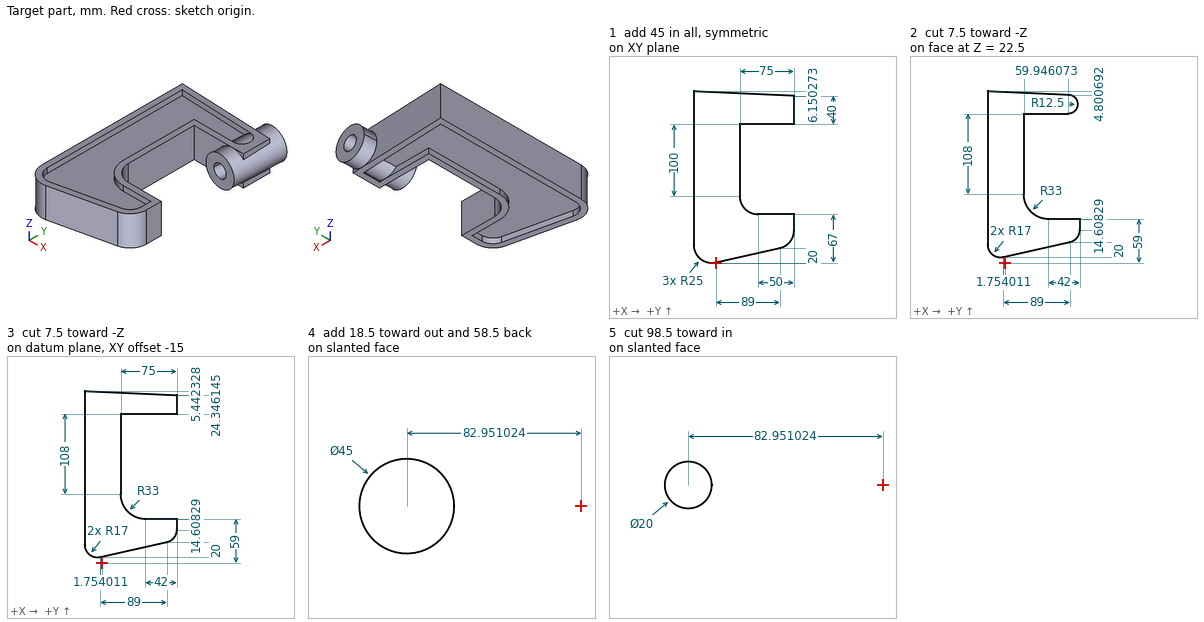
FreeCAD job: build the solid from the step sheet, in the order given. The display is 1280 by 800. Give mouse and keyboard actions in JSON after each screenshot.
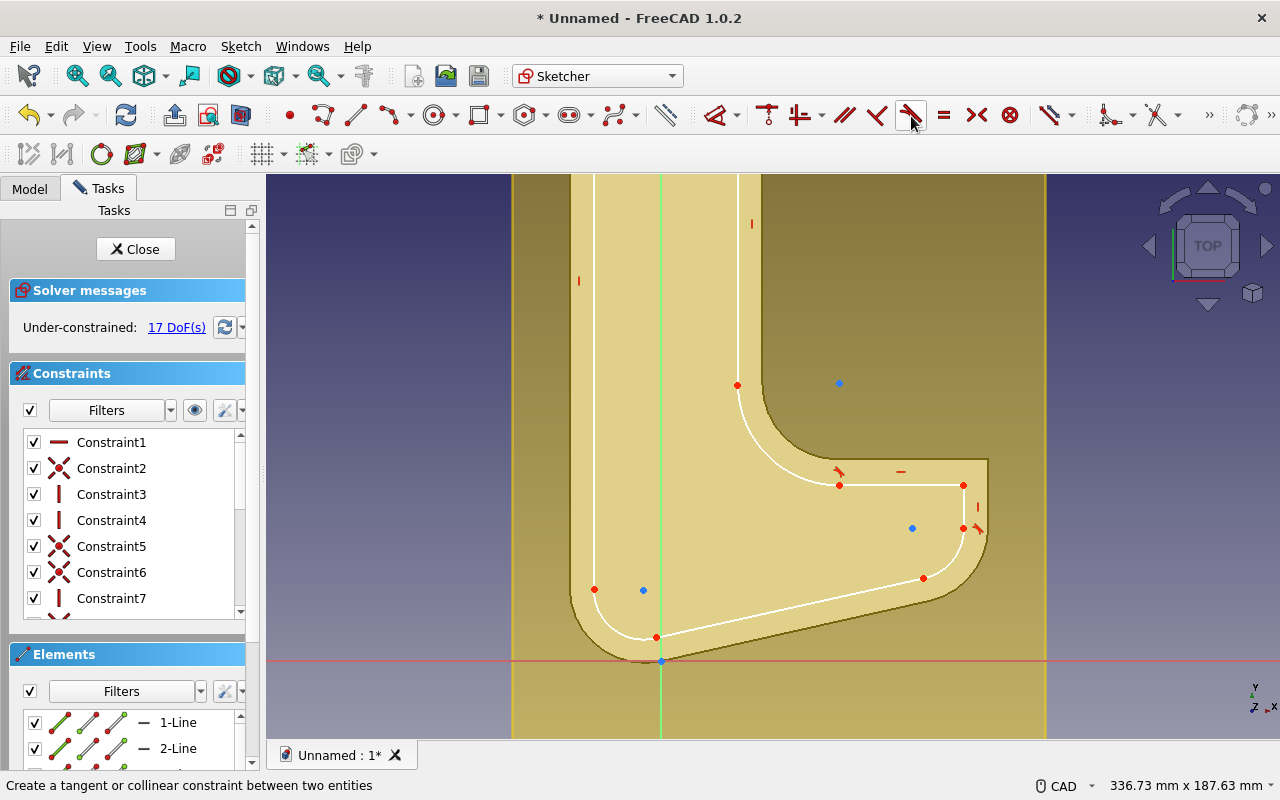
{"action": "left_click", "coordinate": [844, 596]}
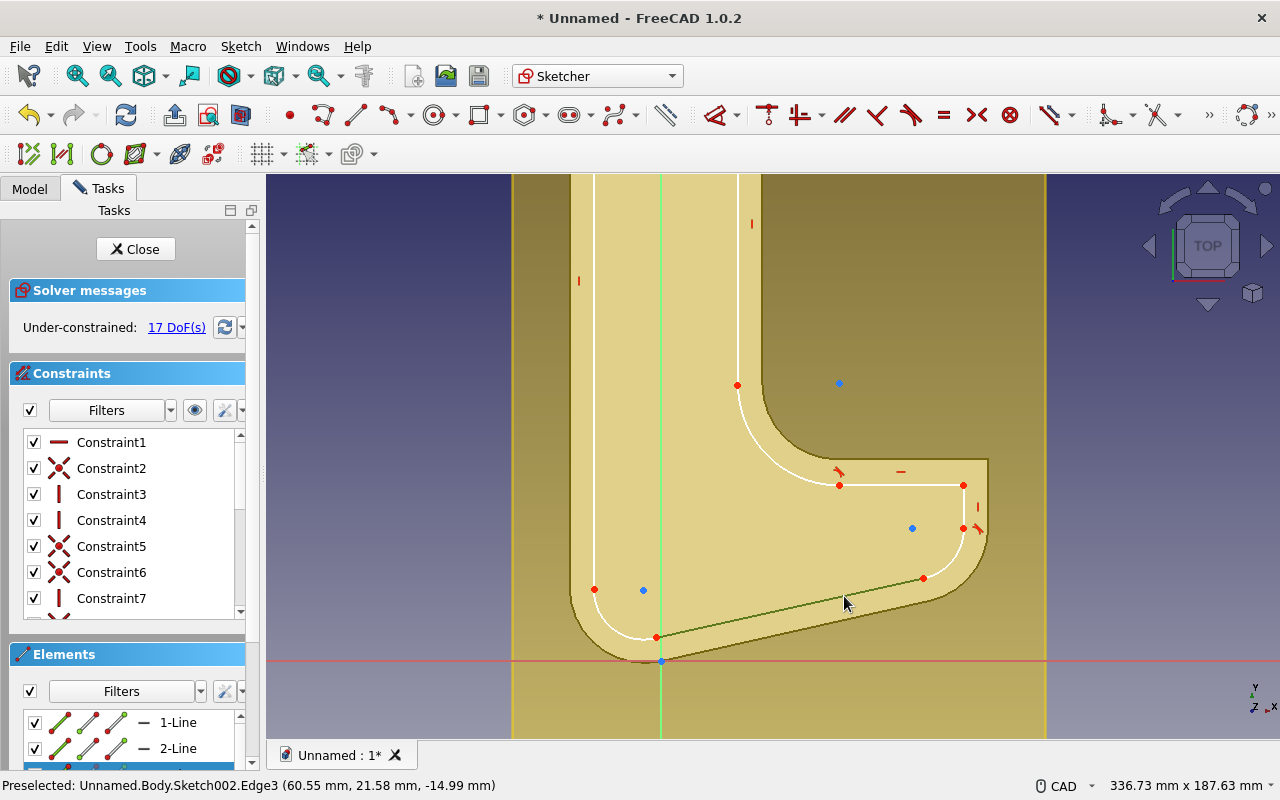
{"action": "left_click", "coordinate": [943, 570]}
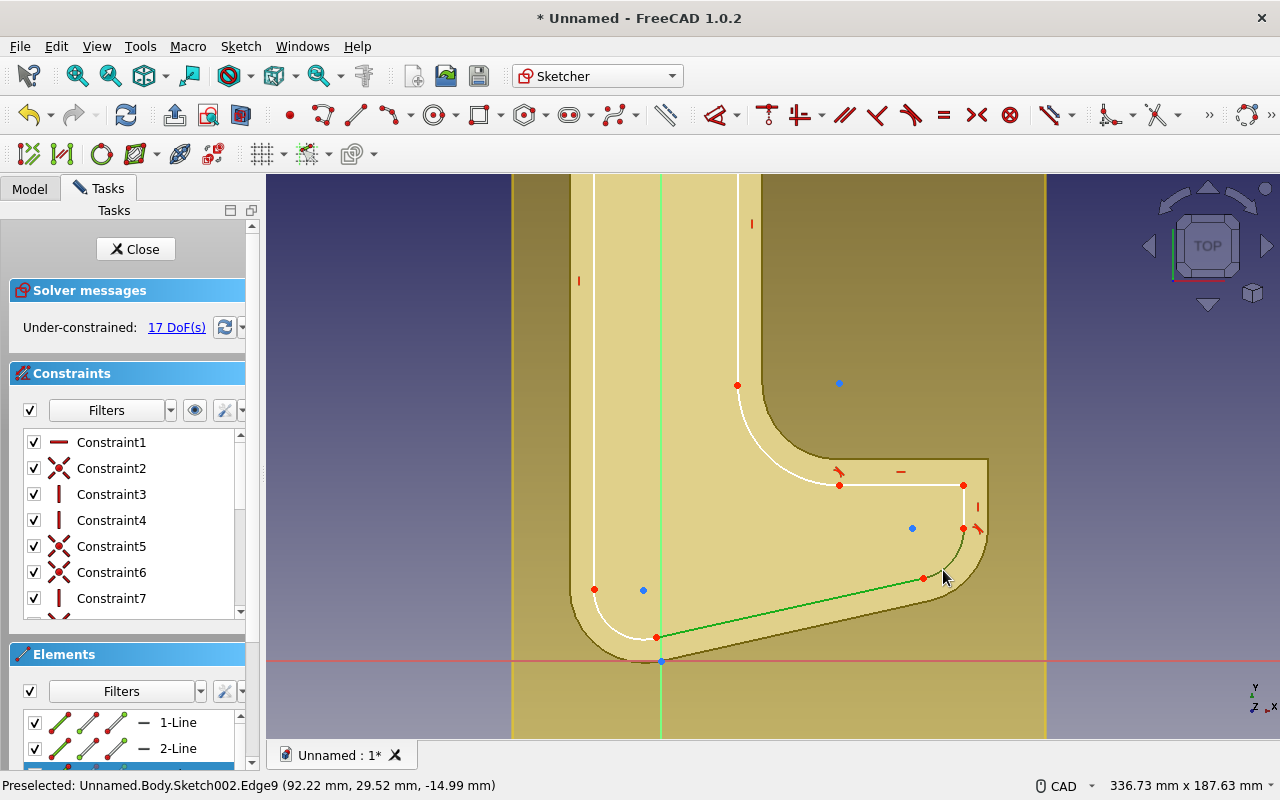
{"action": "left_click", "coordinate": [911, 116]}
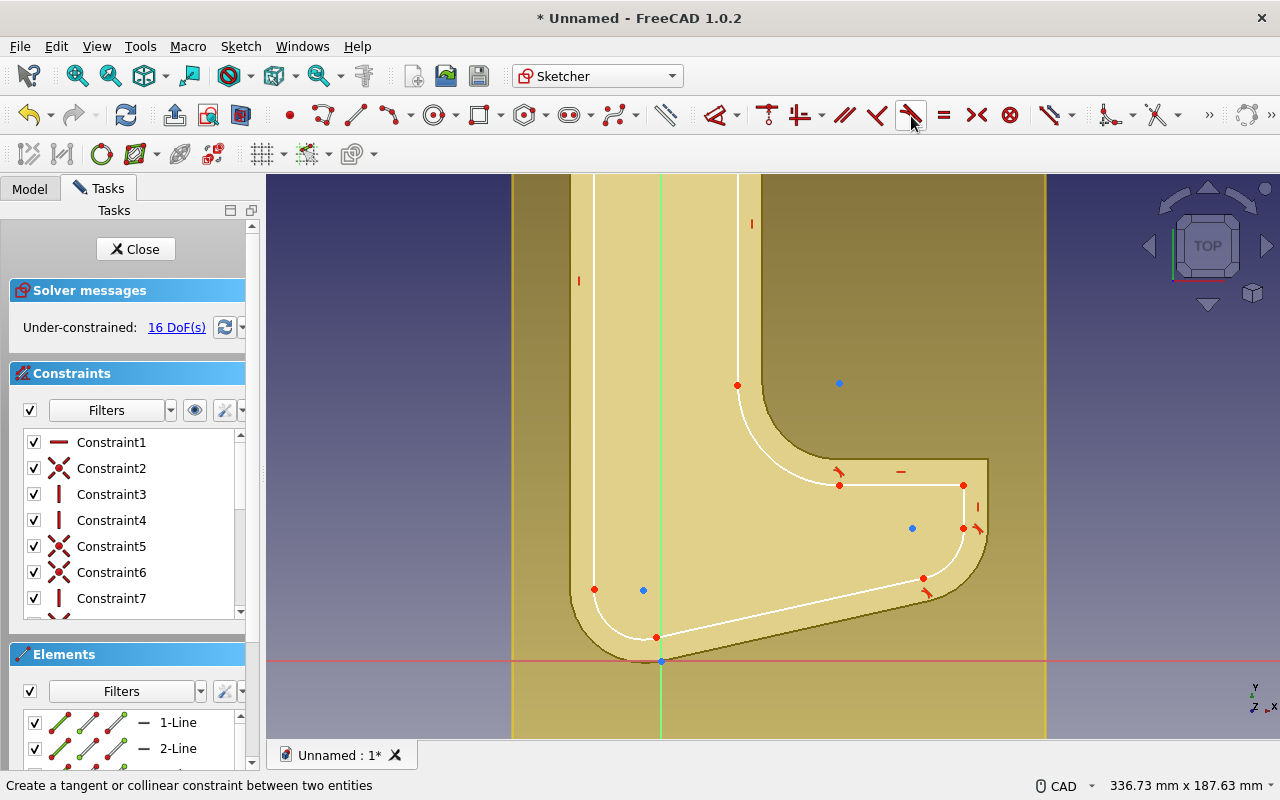
{"action": "left_click", "coordinate": [844, 596]}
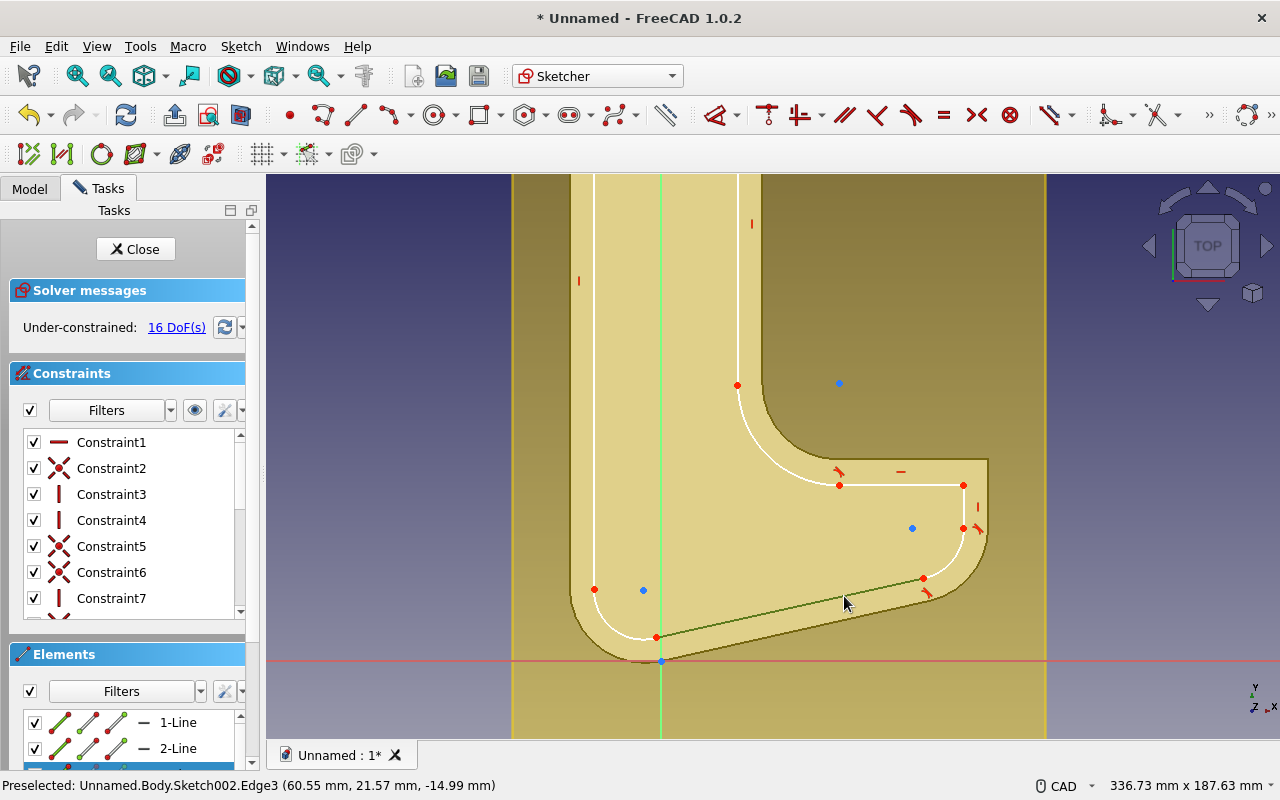
{"action": "left_click", "coordinate": [601, 616]}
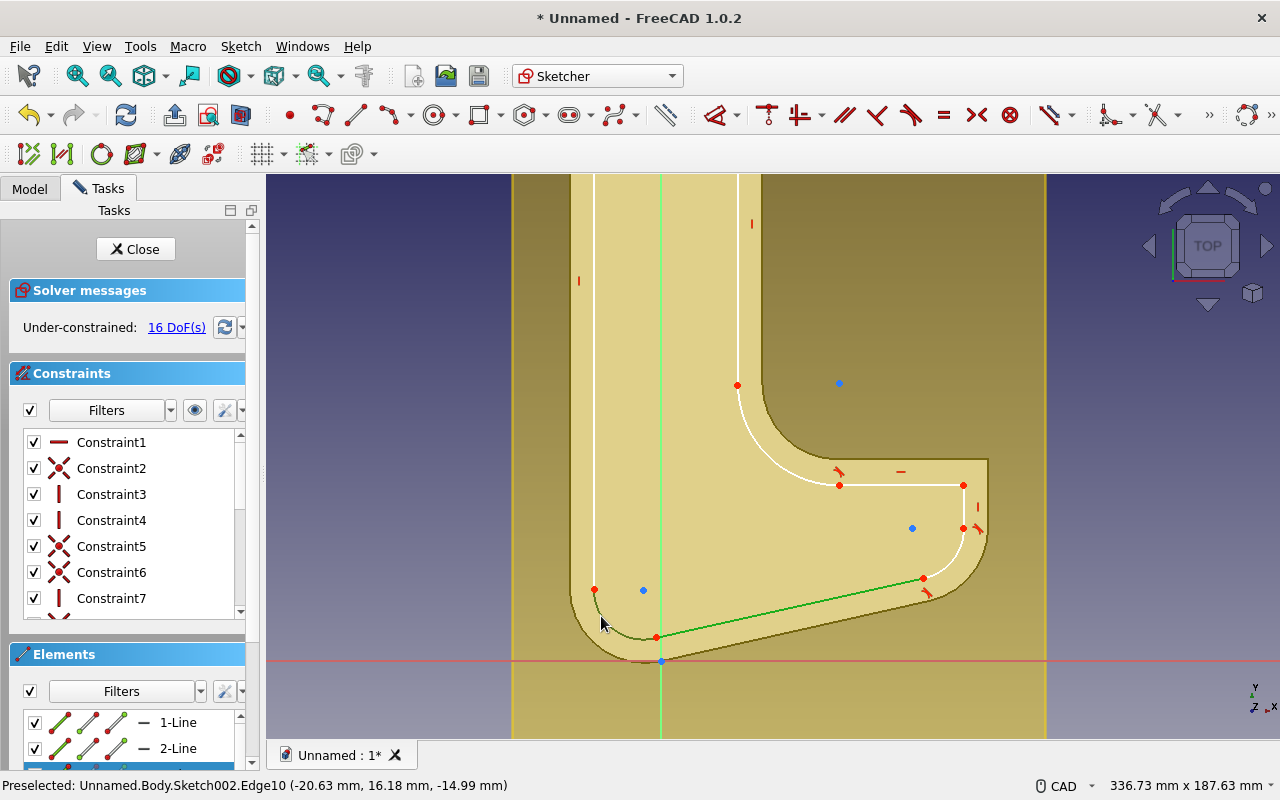
{"action": "left_click", "coordinate": [911, 116]}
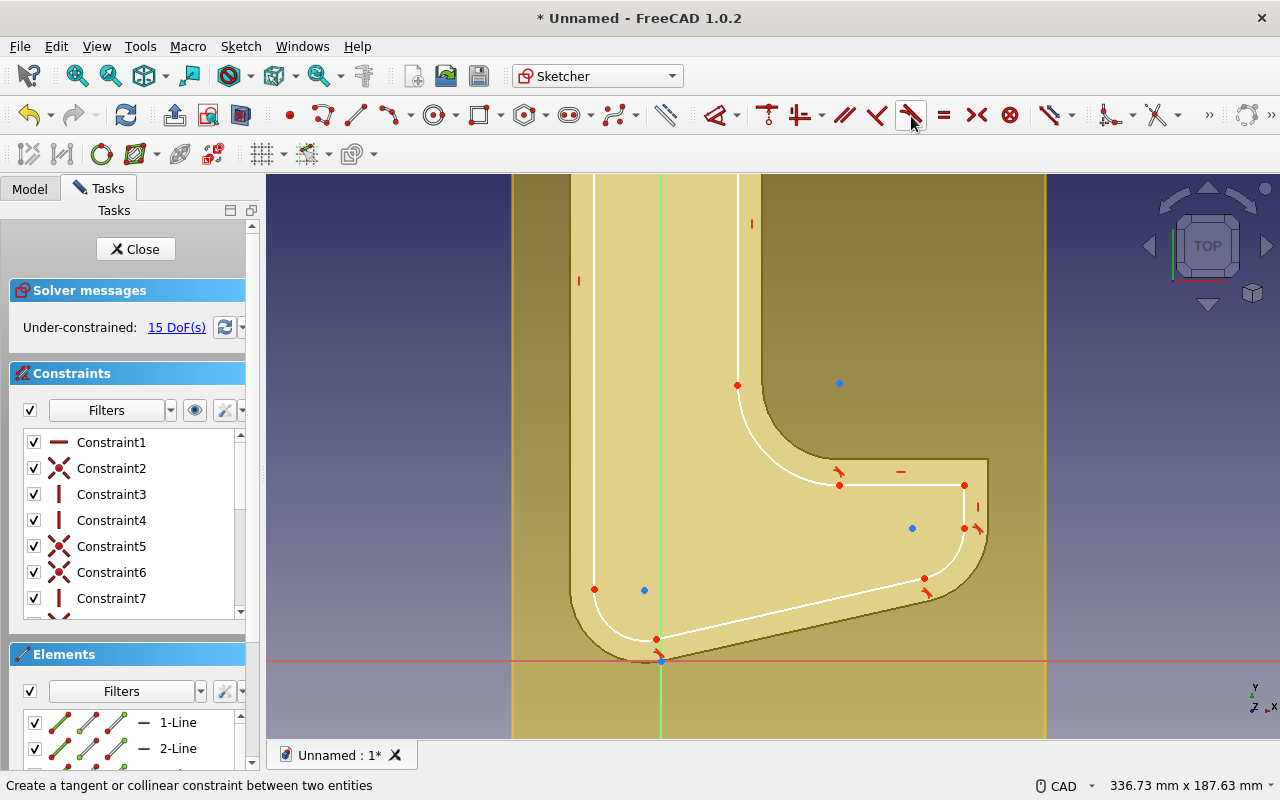
{"action": "left_click", "coordinate": [594, 404]}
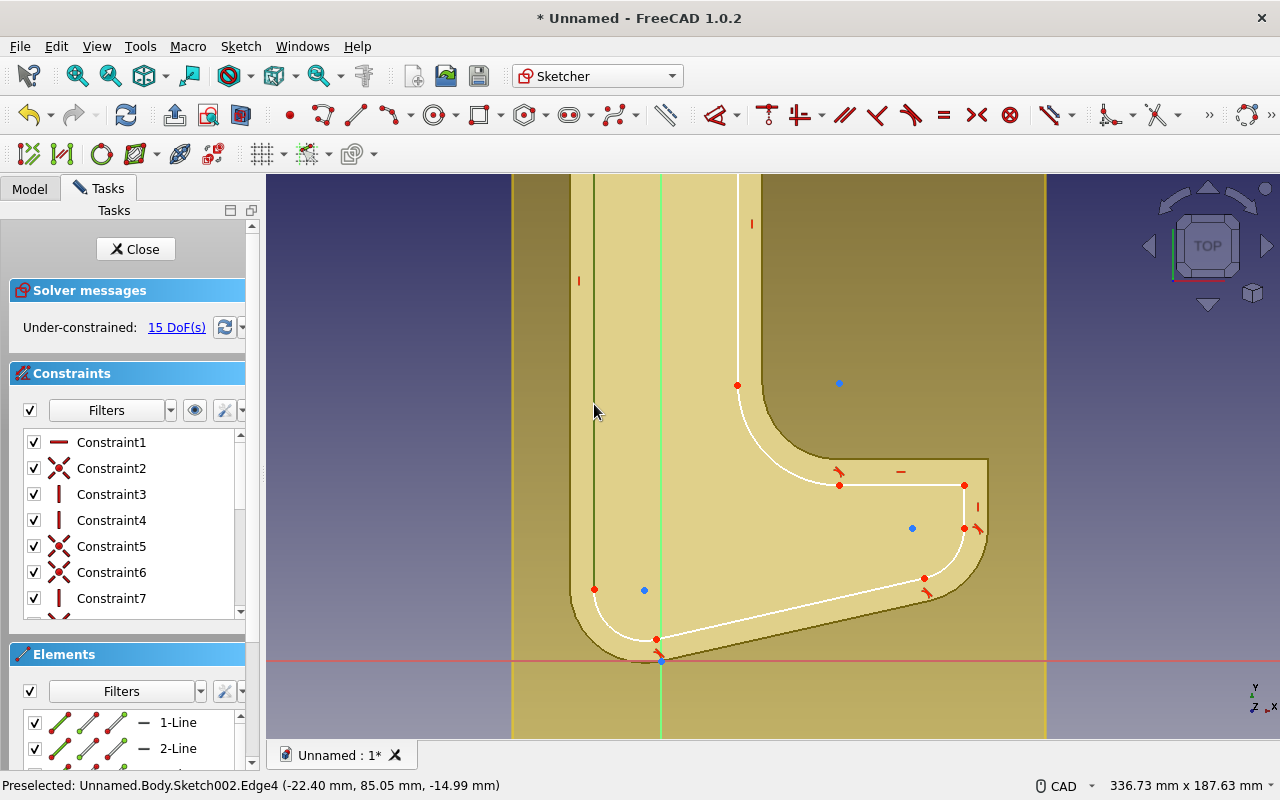
{"action": "left_click", "coordinate": [601, 616]}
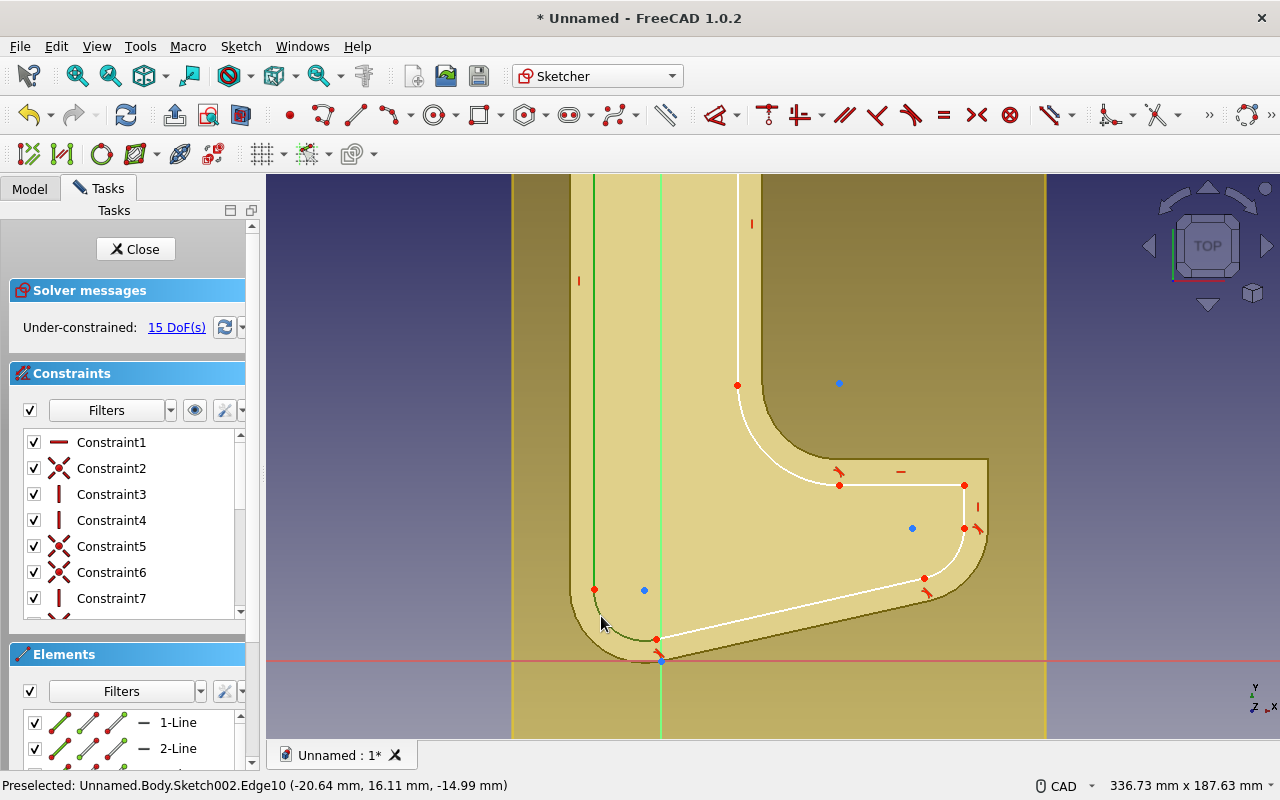
{"action": "left_click", "coordinate": [911, 116]}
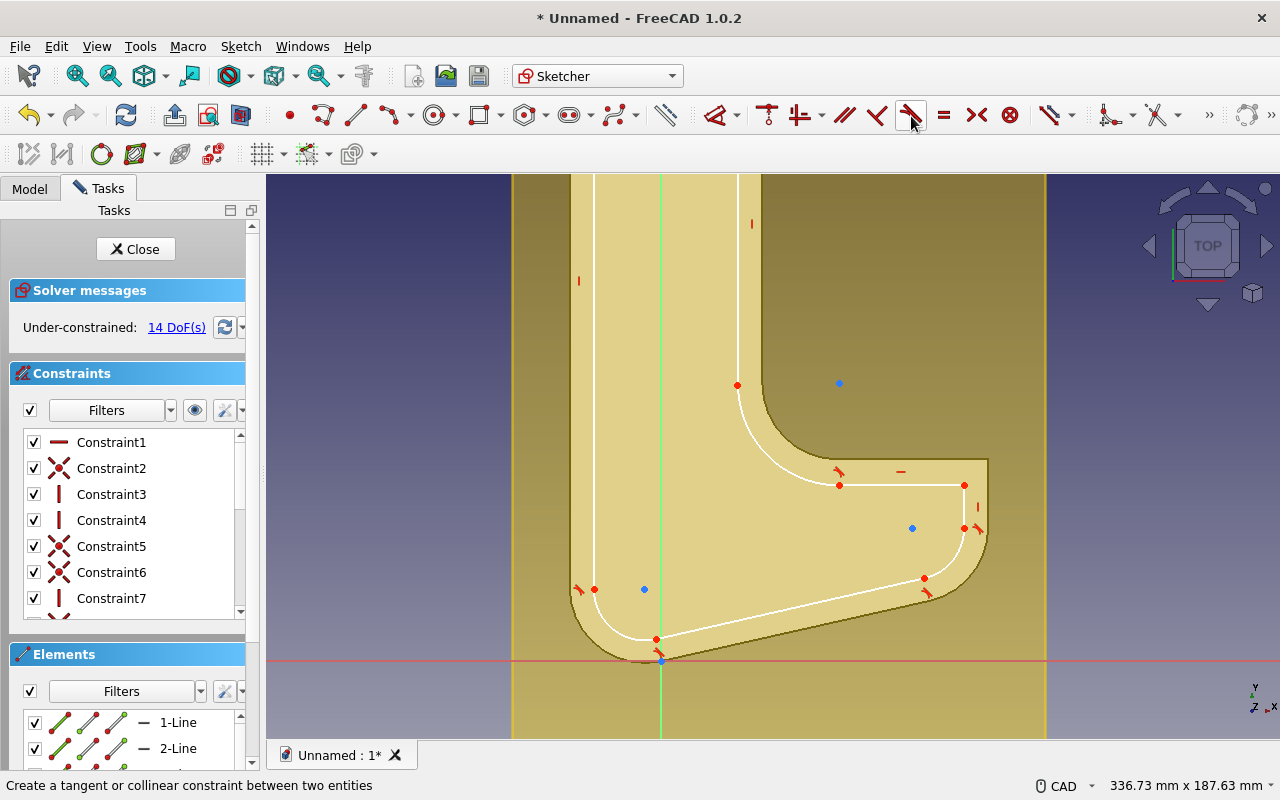
{"action": "left_click", "coordinate": [738, 288]}